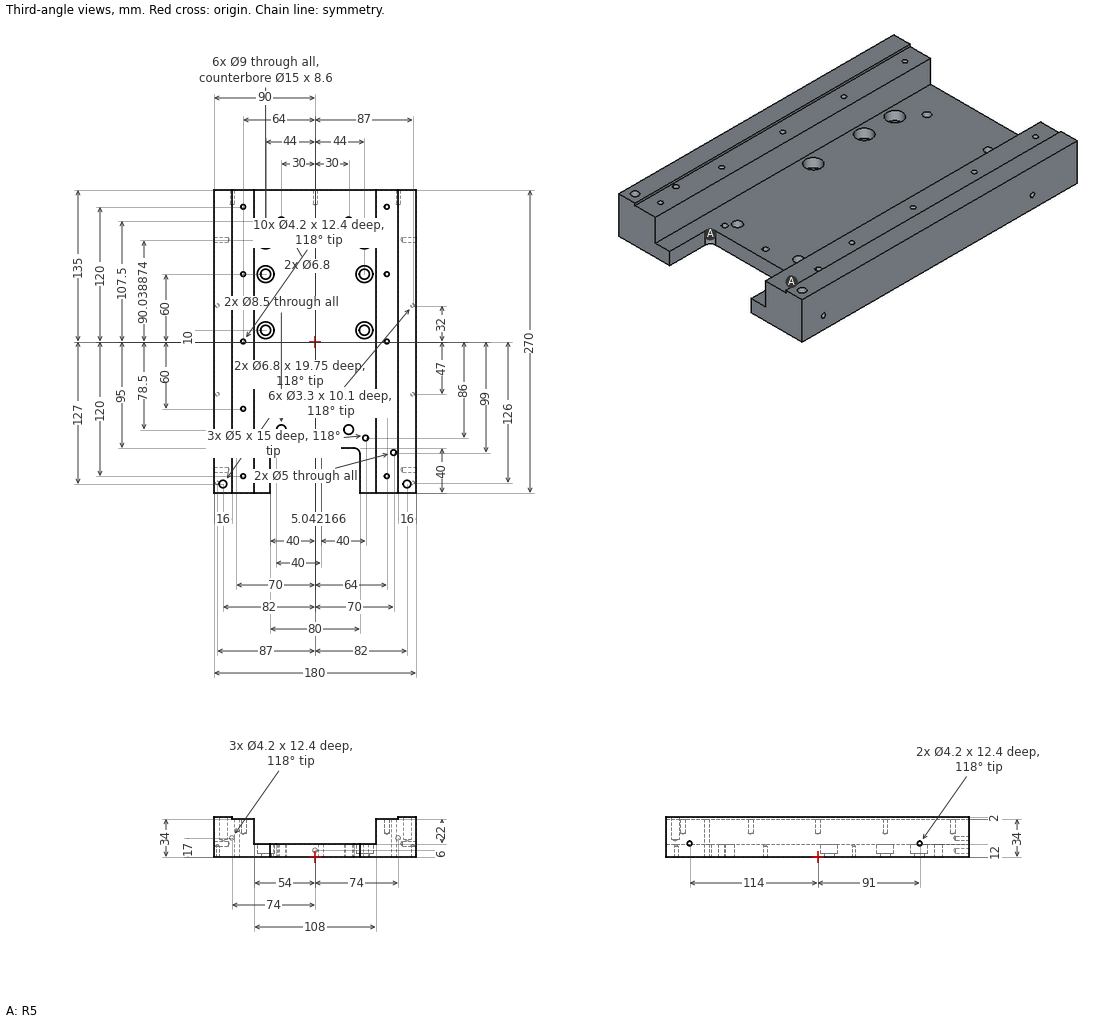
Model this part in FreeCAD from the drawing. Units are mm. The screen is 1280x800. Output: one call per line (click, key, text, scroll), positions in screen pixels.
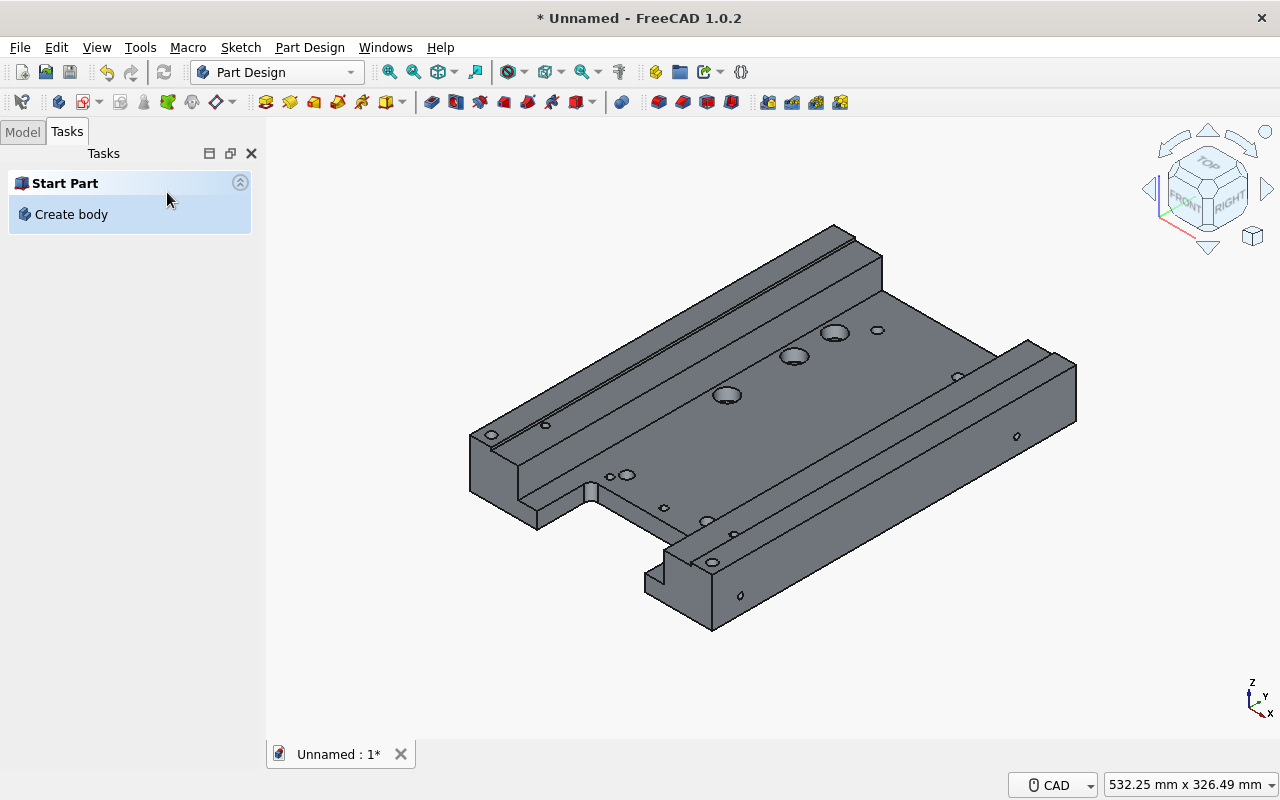
click(843, 262)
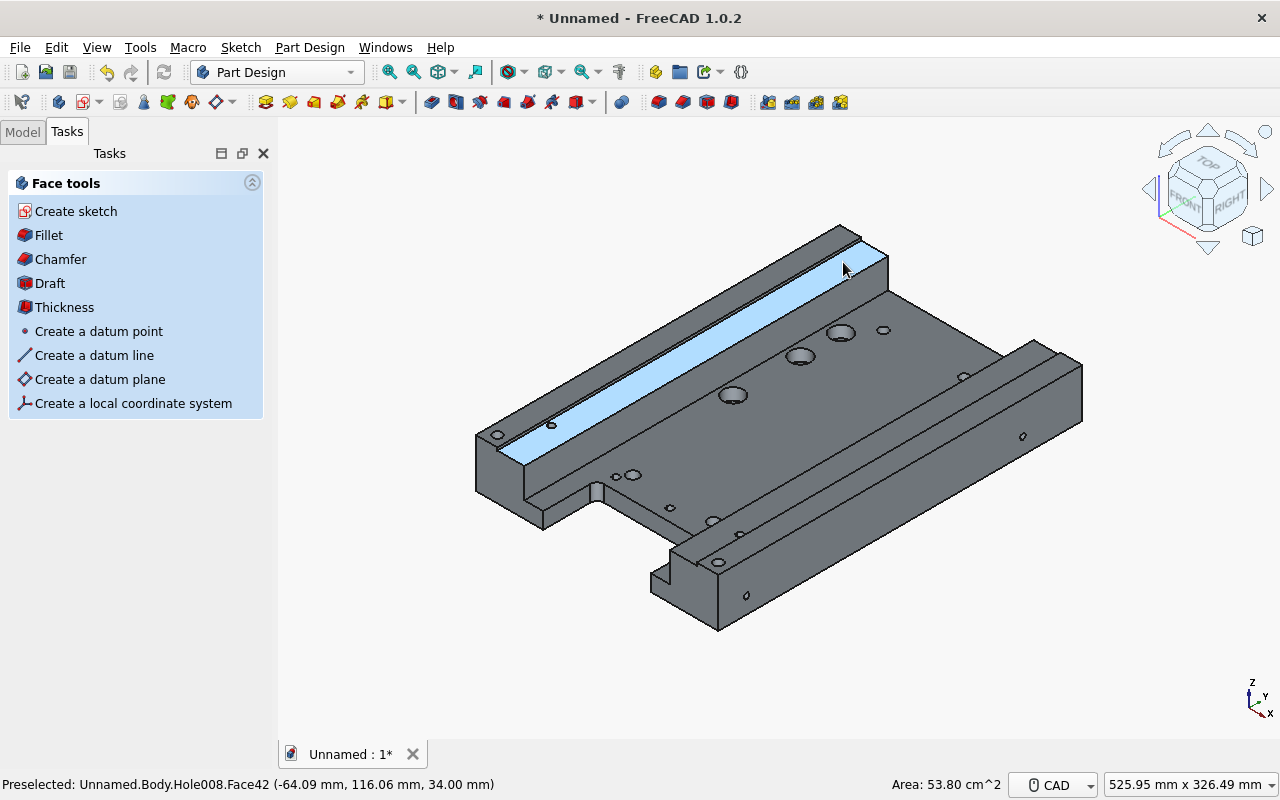
click(84, 102)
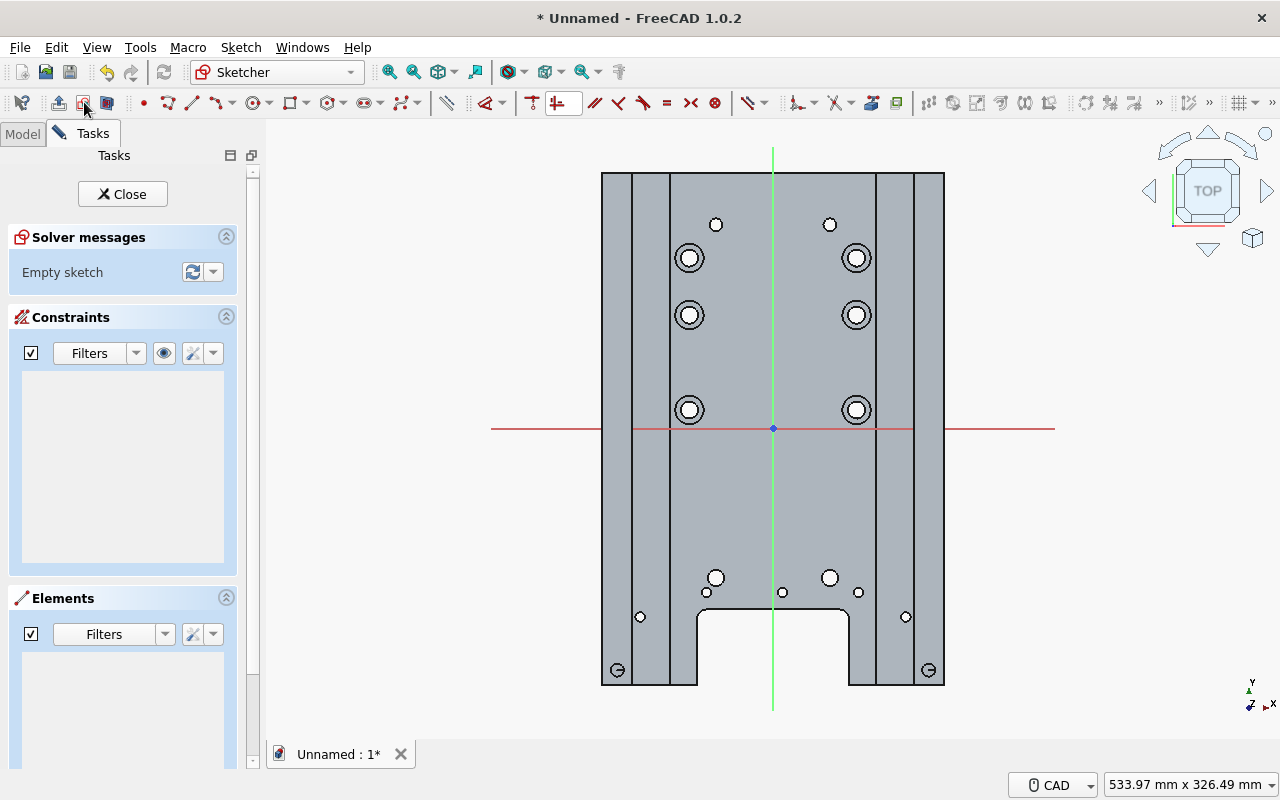
click(254, 104)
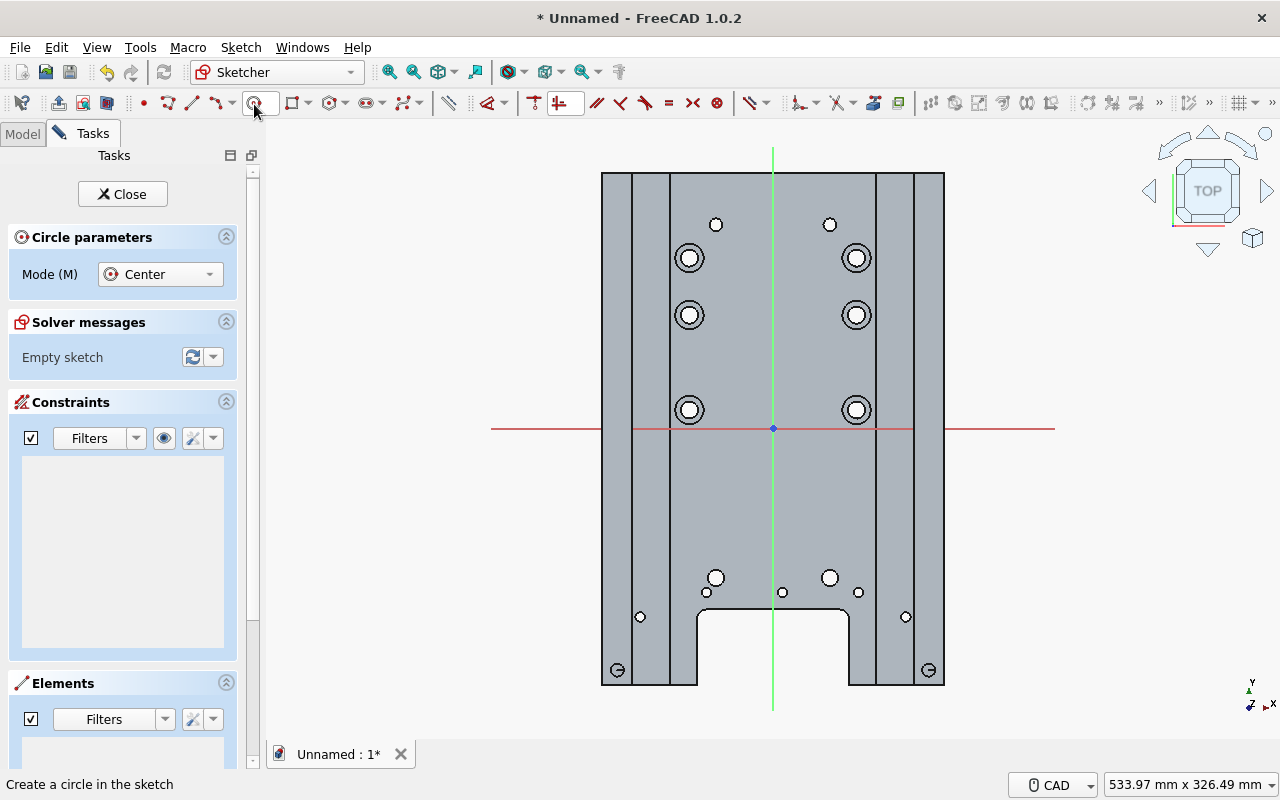
scroll(651, 429, up, 9)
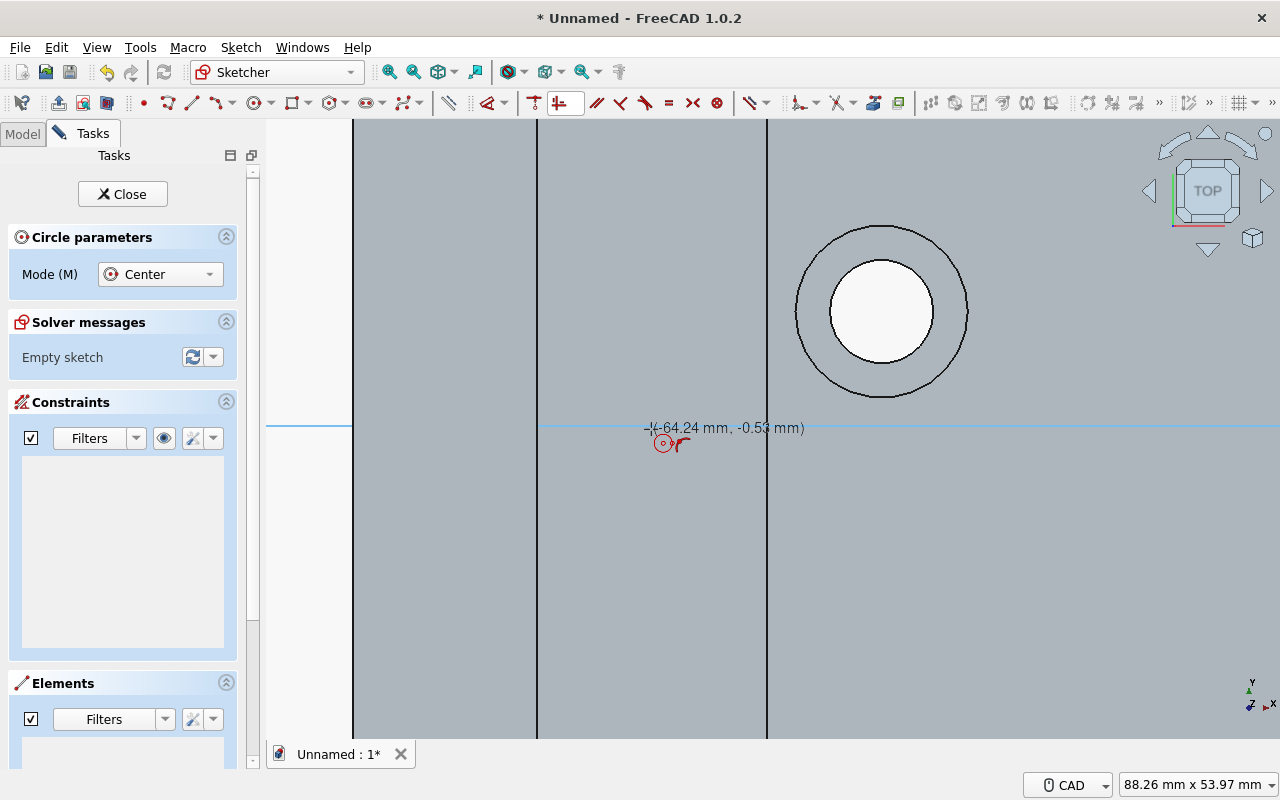
scroll(598, 429, down, 10)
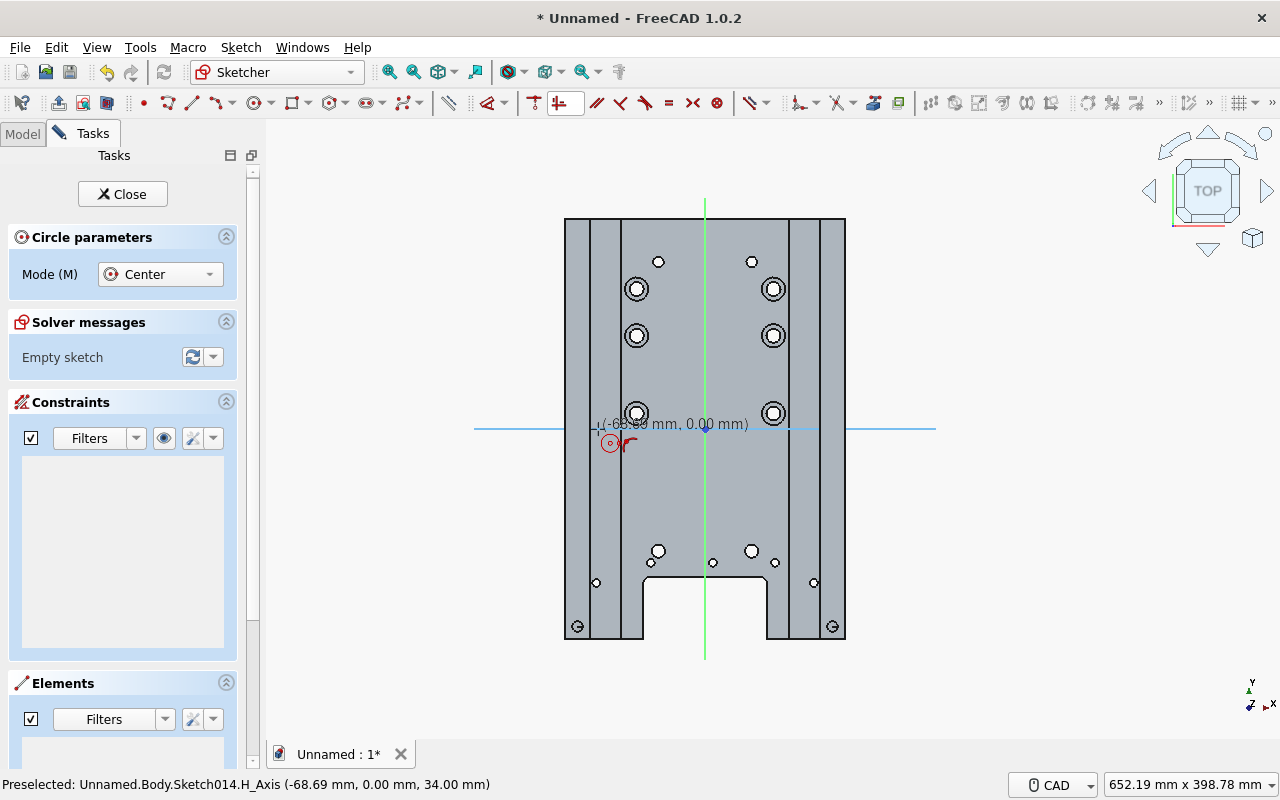
click(606, 429)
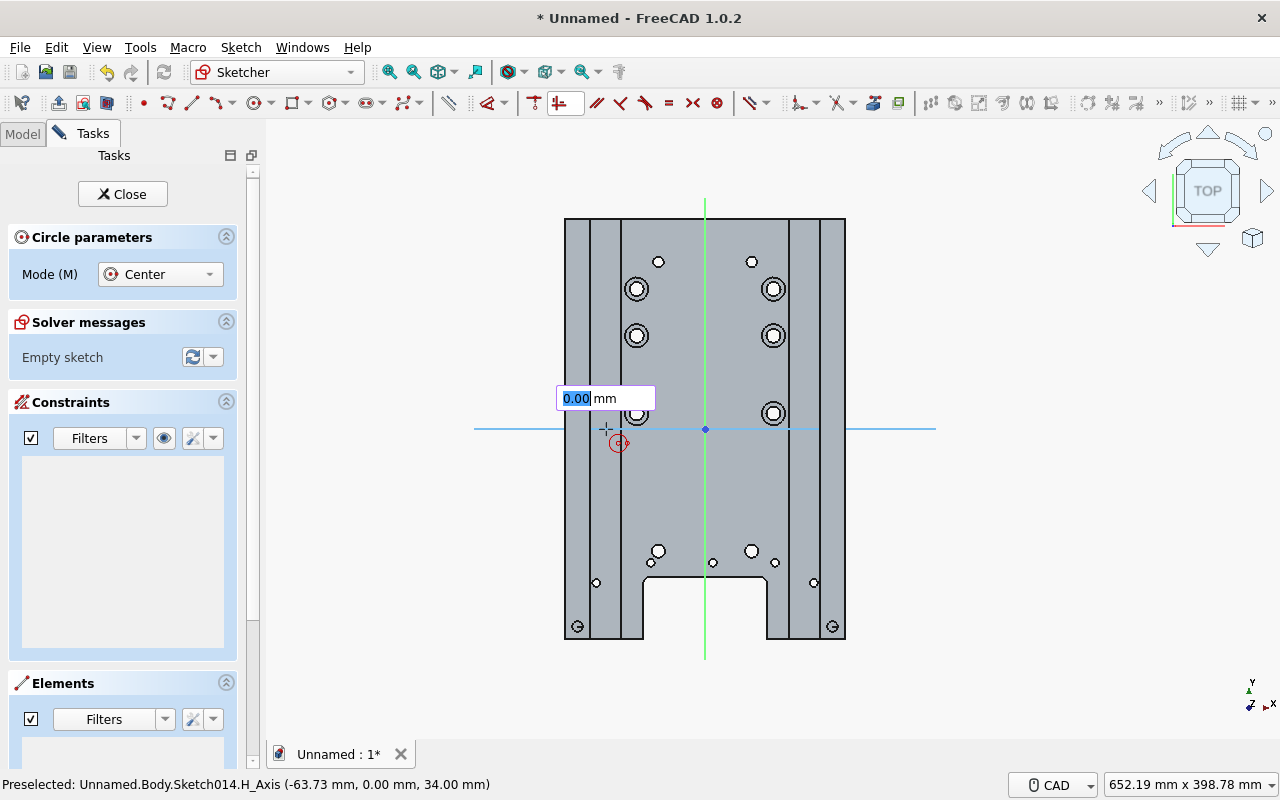
scroll(607, 426, up, 9)
move(603, 424)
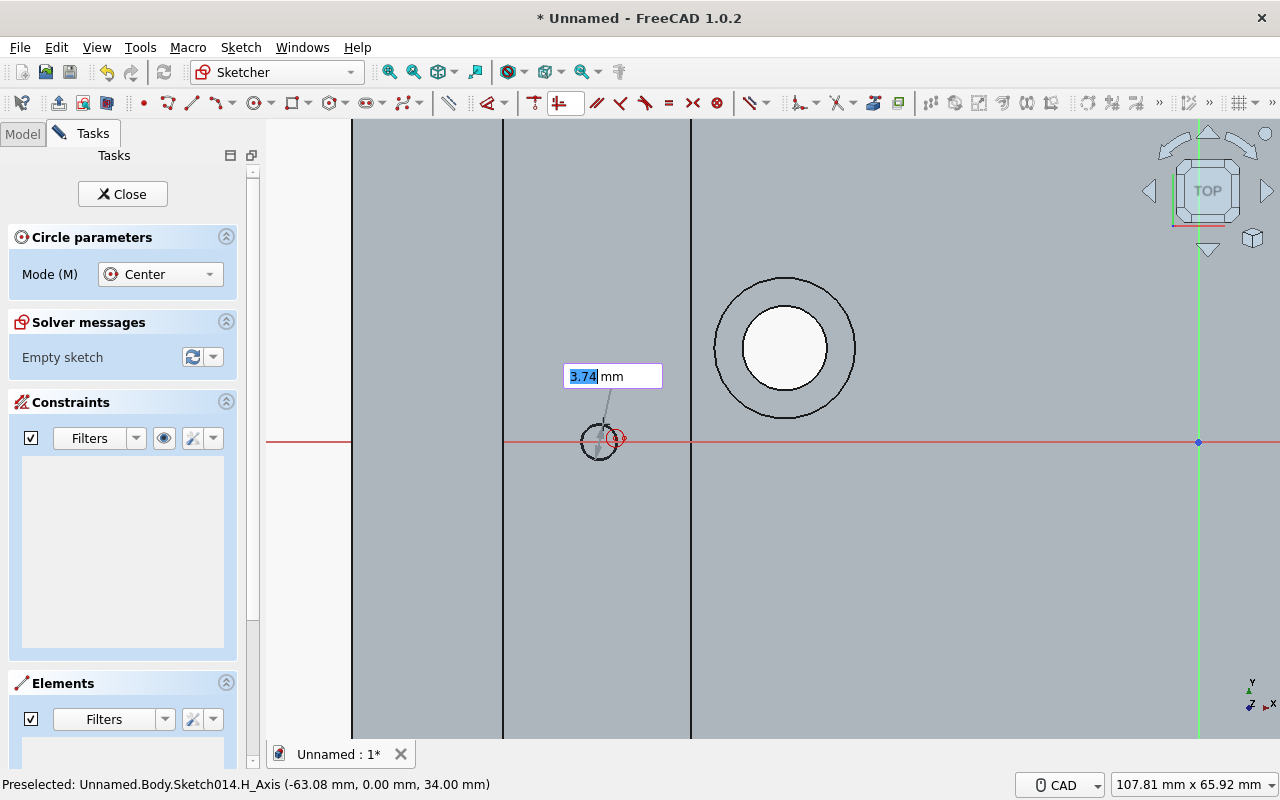
text(4.2)
key(Return)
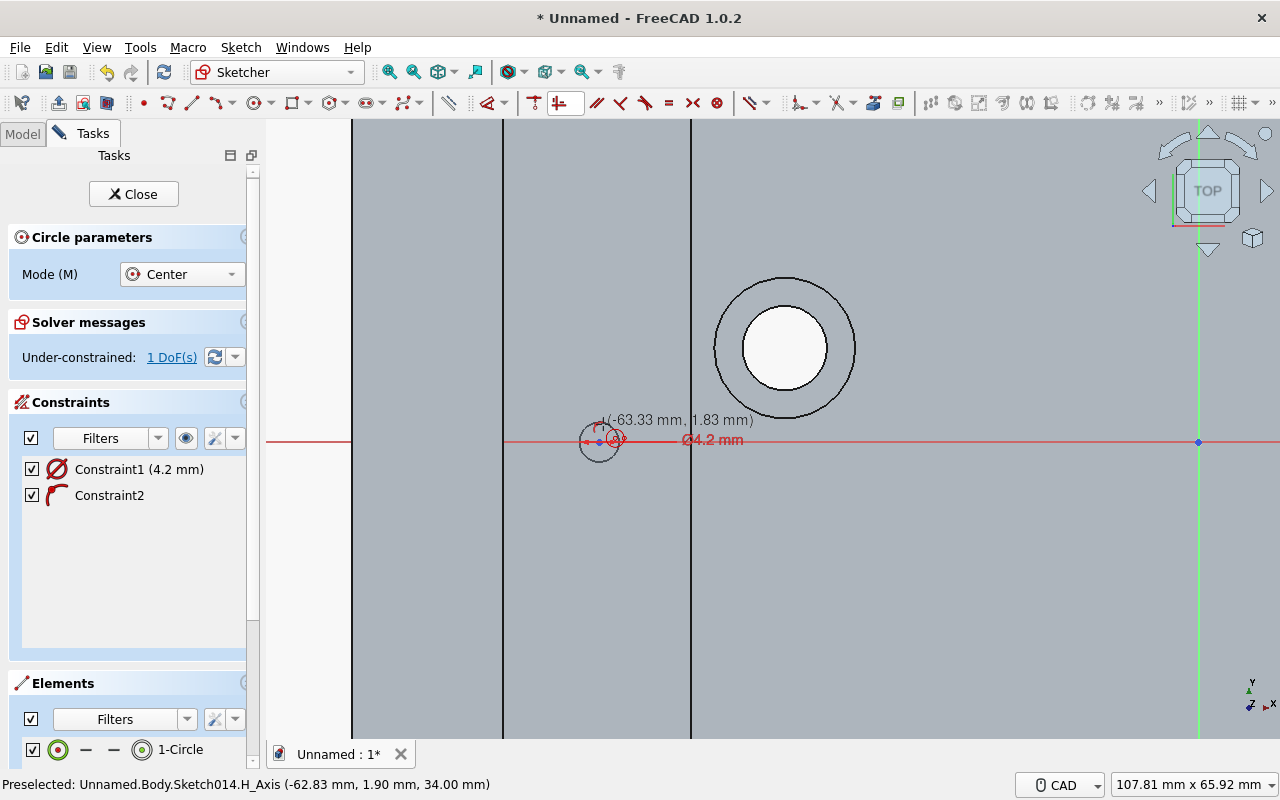
scroll(607, 426, down, 9)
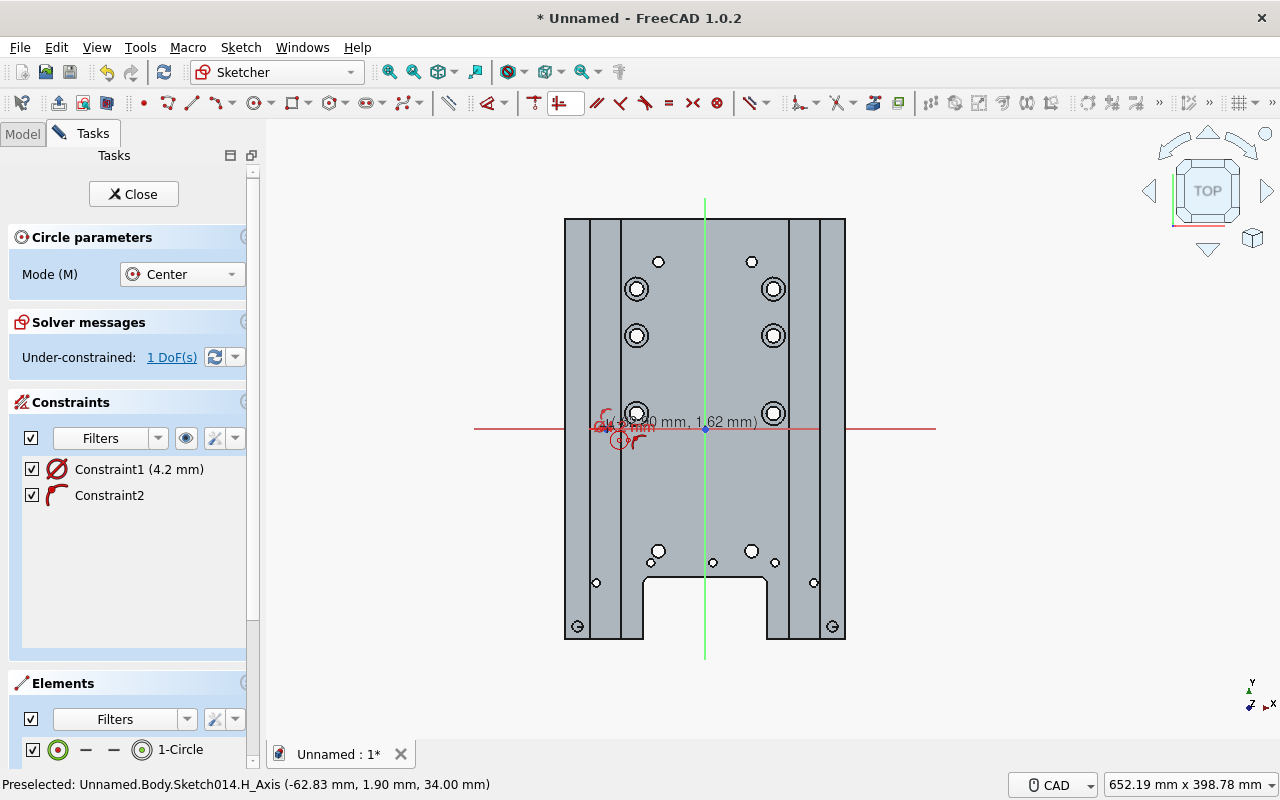
scroll(606, 336, up, 10)